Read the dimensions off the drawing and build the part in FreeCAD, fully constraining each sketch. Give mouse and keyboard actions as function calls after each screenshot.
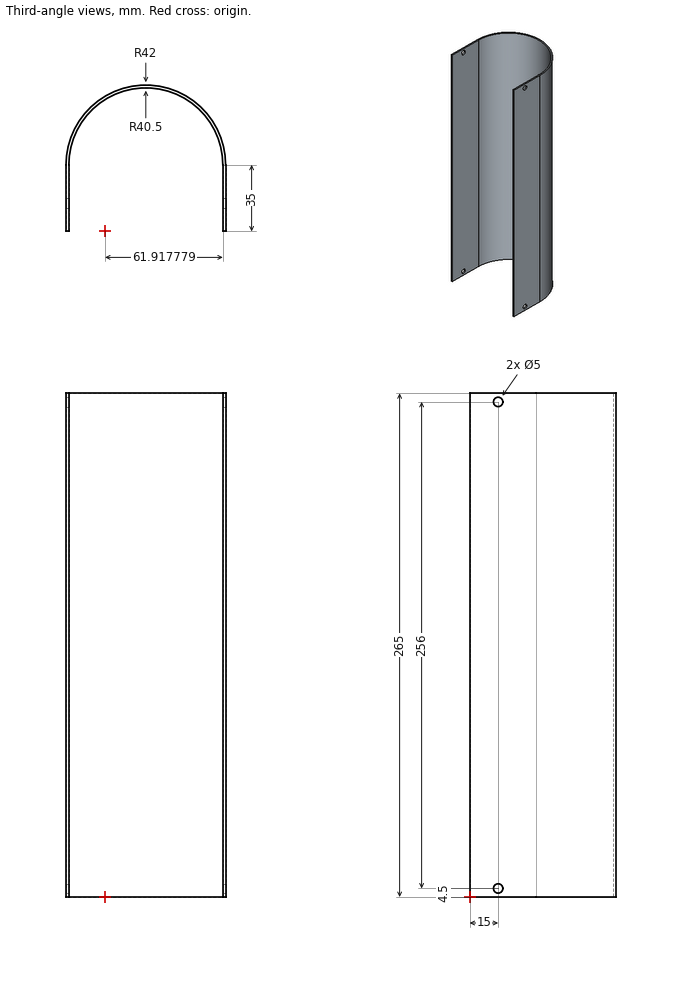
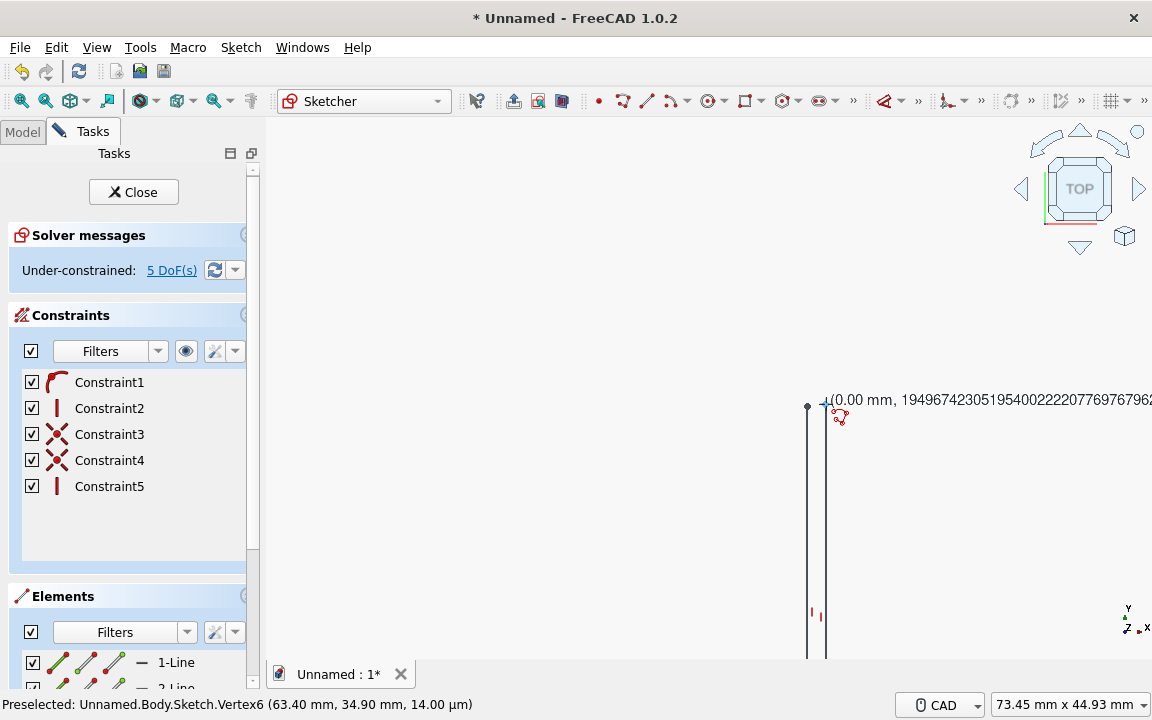
scroll(827, 403, down, 5)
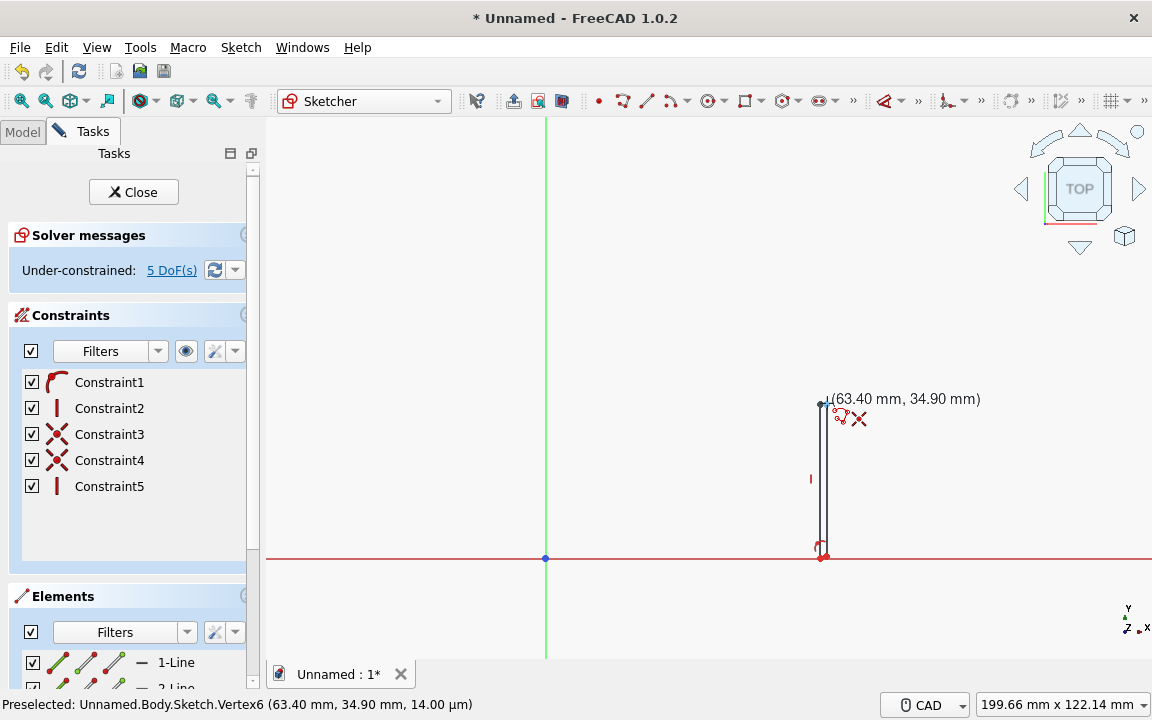
click(454, 404)
click(454, 559)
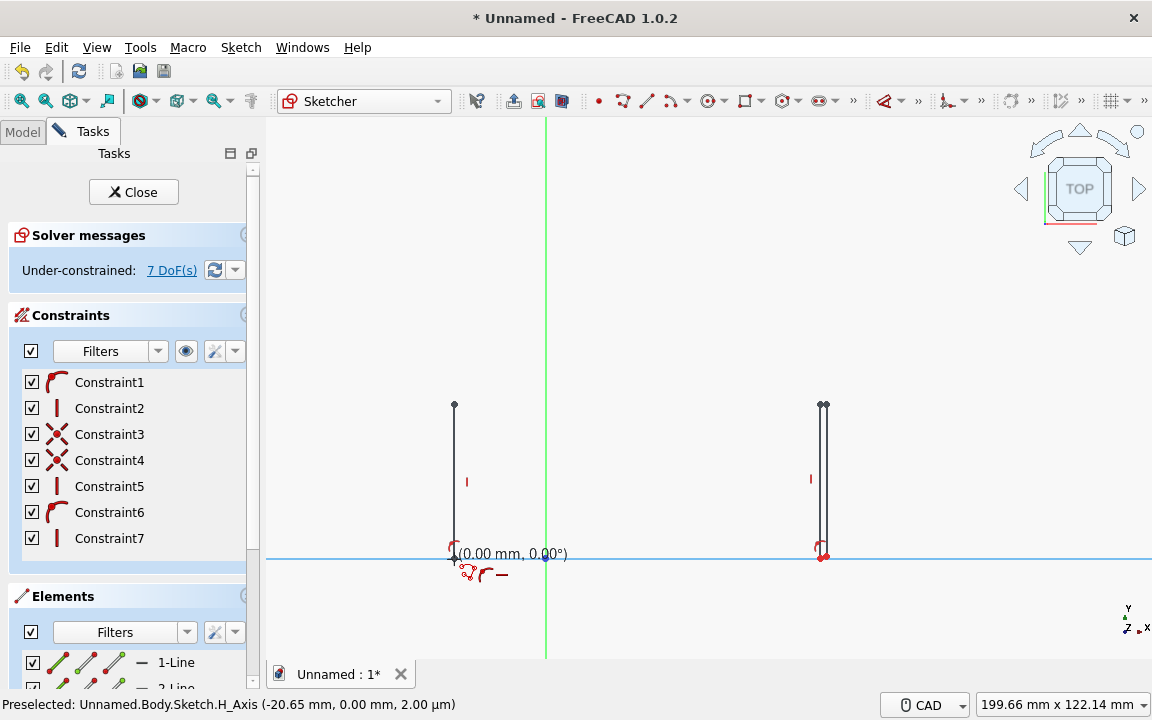
scroll(461, 559, up, 5)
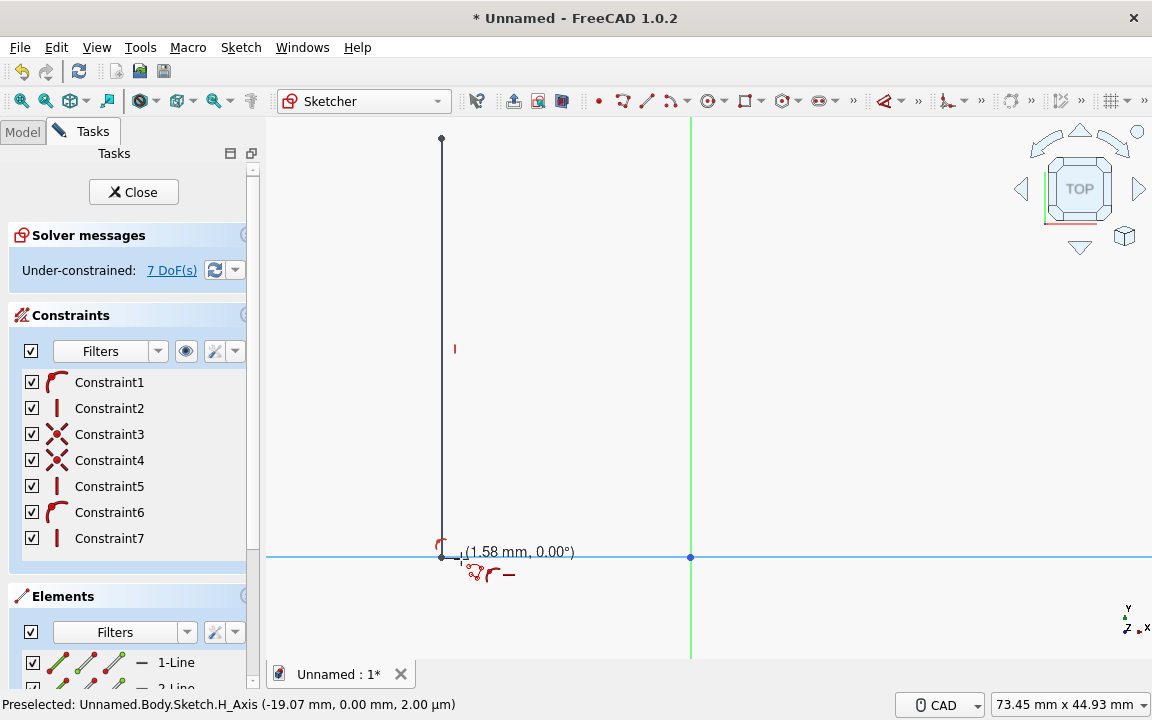
click(461, 548)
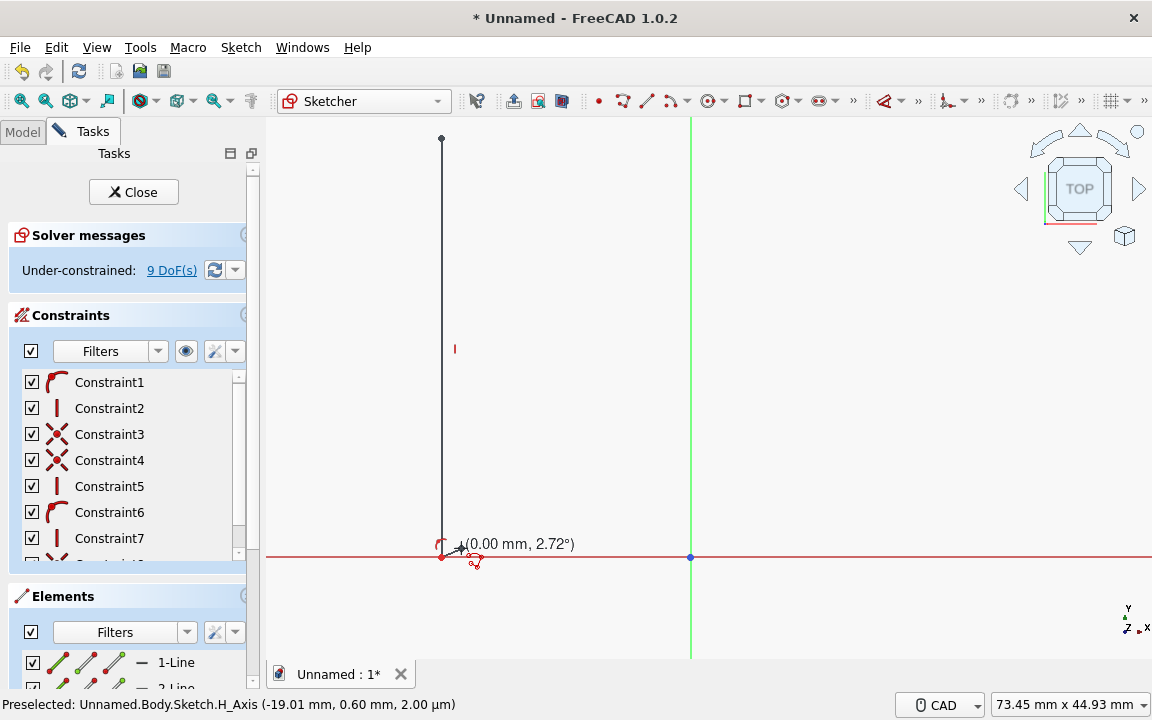
scroll(461, 560, down, 5)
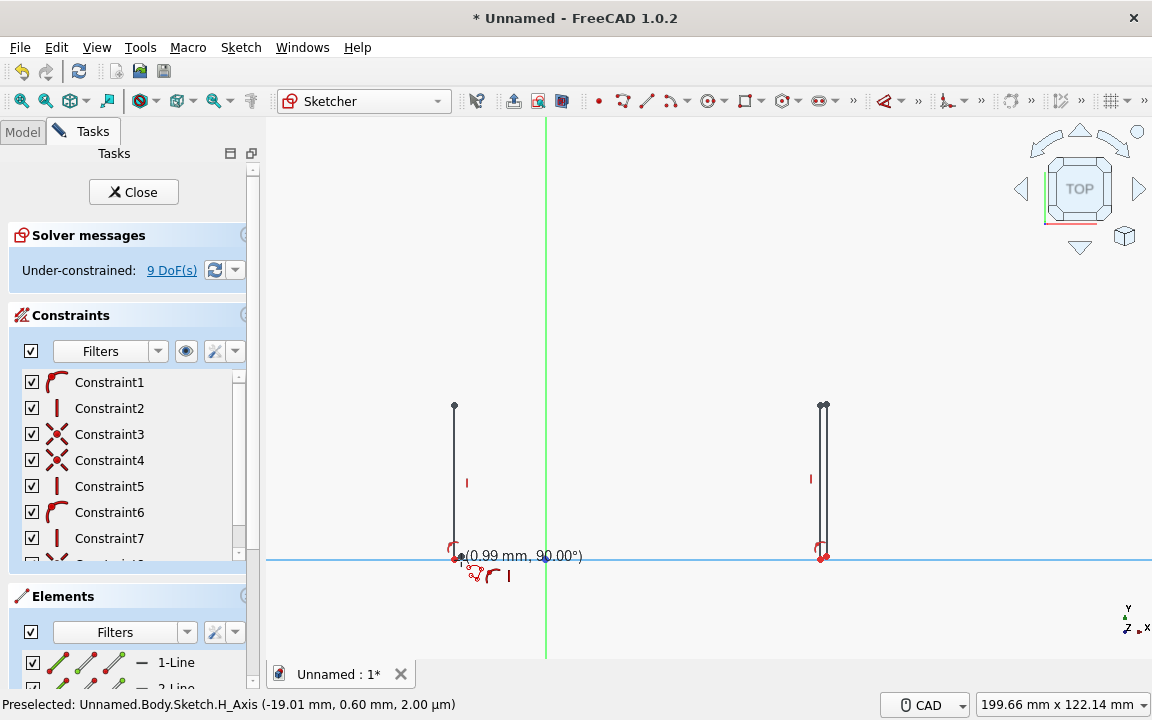
scroll(461, 404, up, 5)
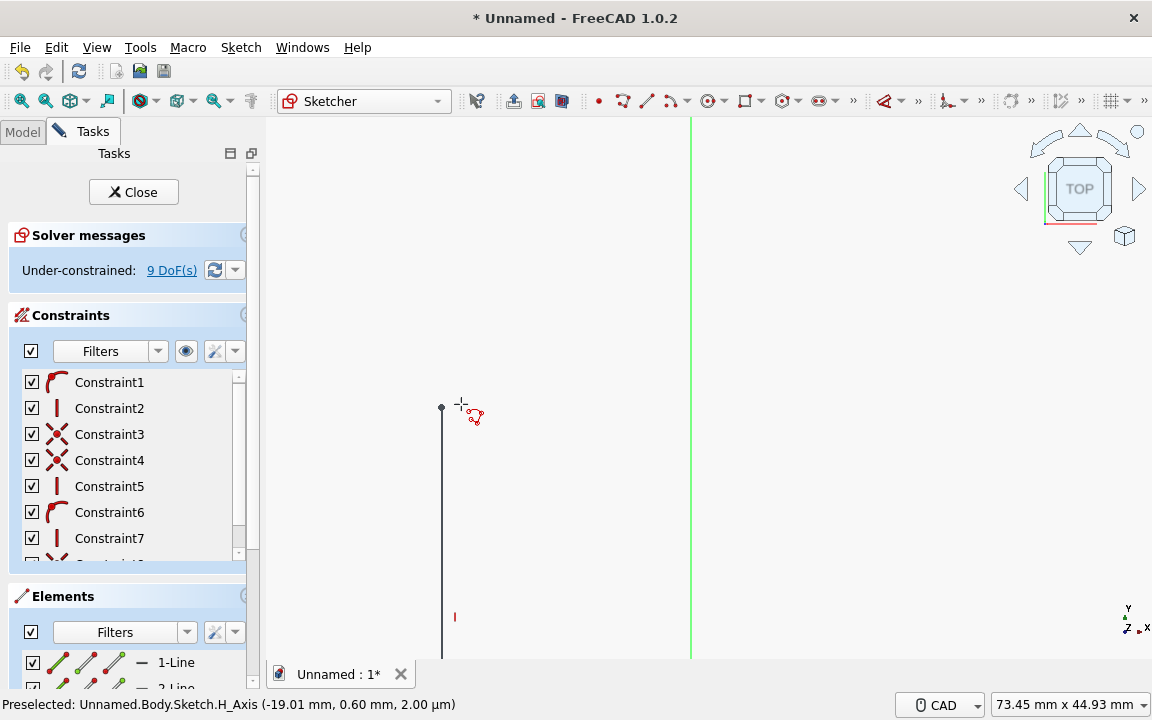
click(461, 404)
right_click(461, 404)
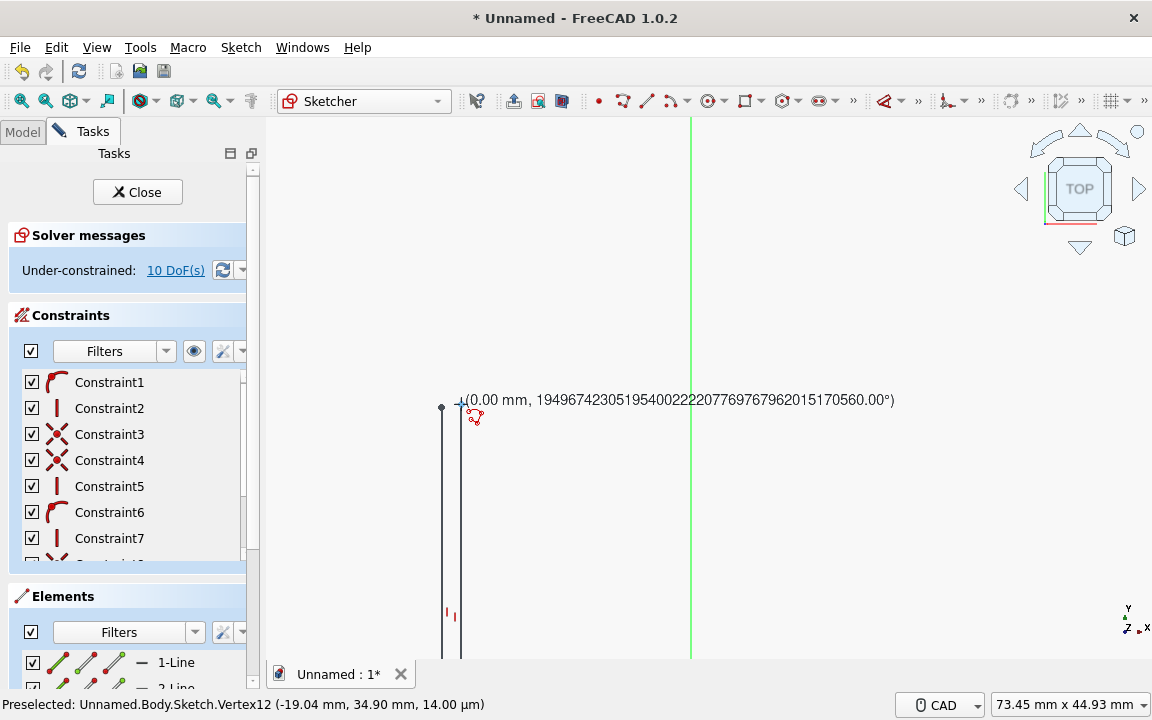
key(g)
key(3)
key(a)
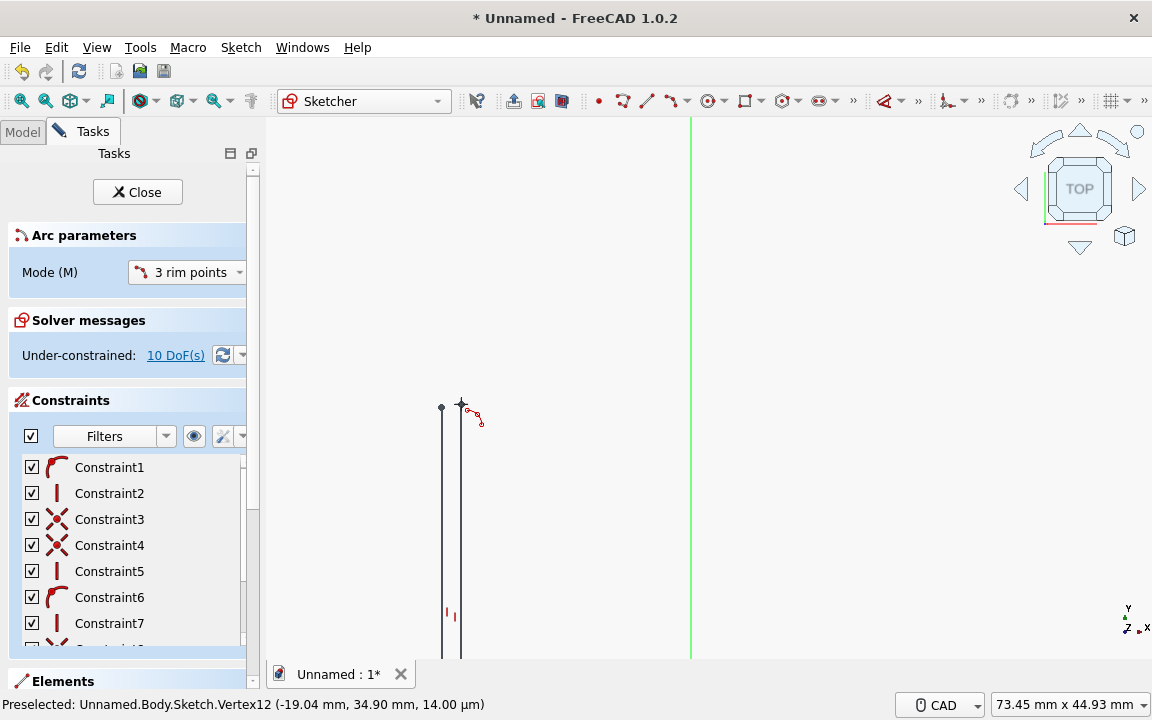
scroll(461, 403, down, 5)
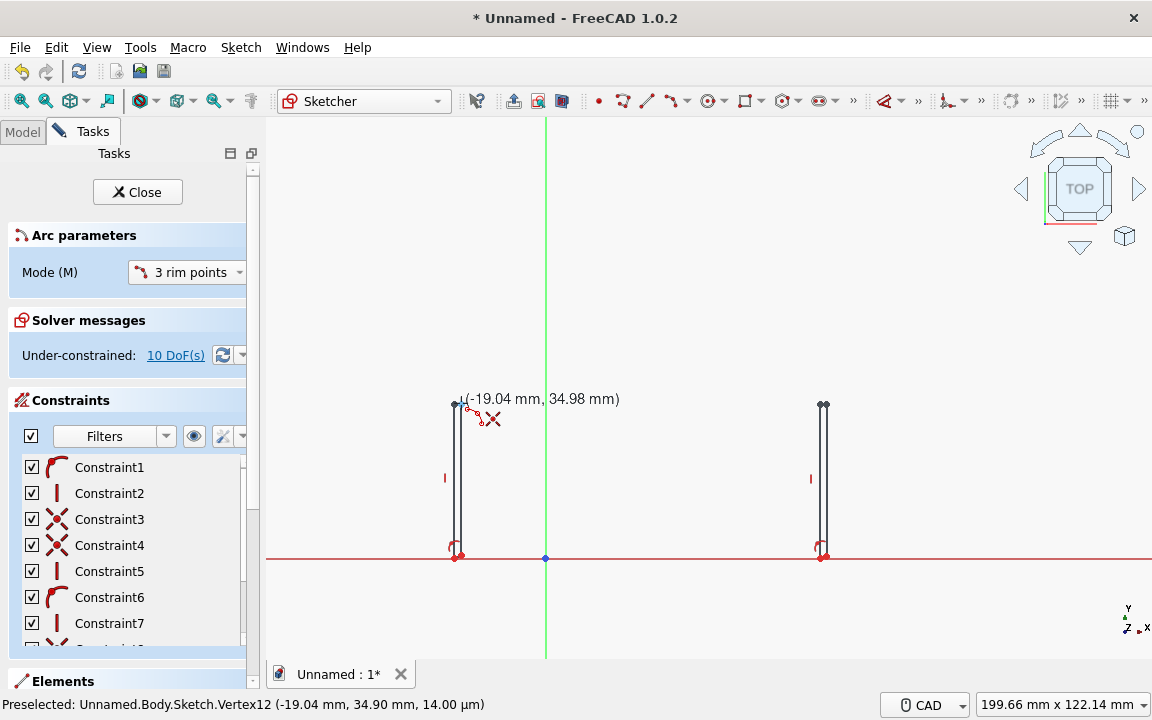
scroll(827, 404, up, 5)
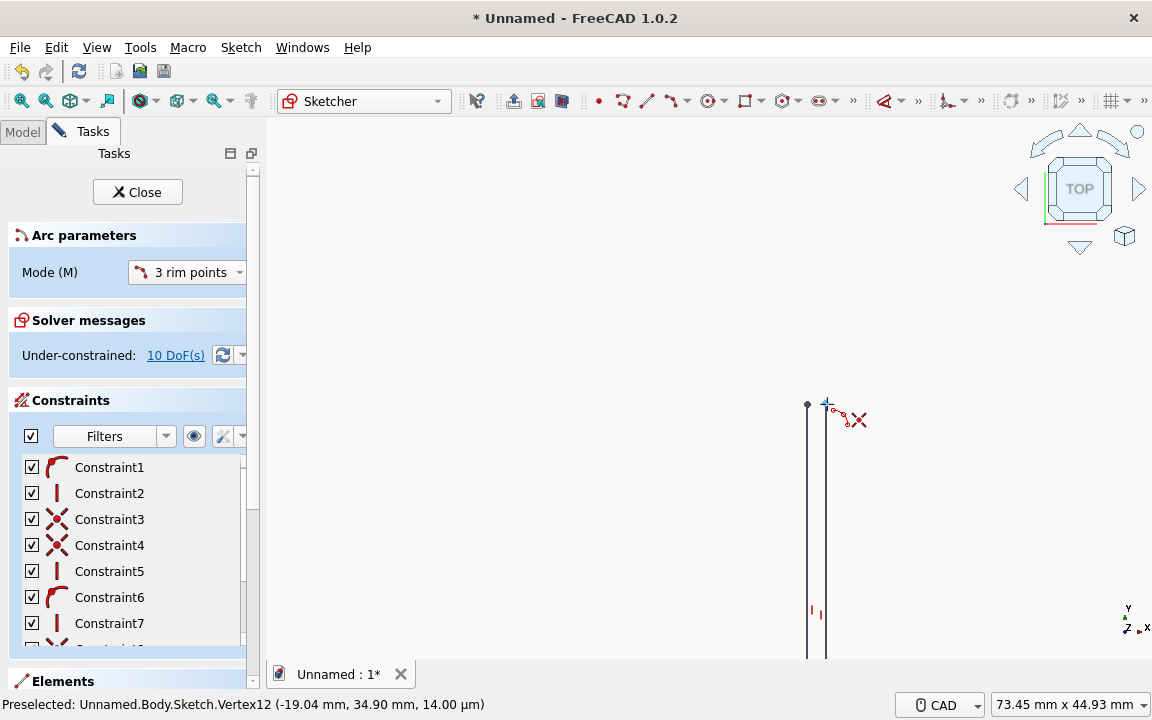
click(826, 403)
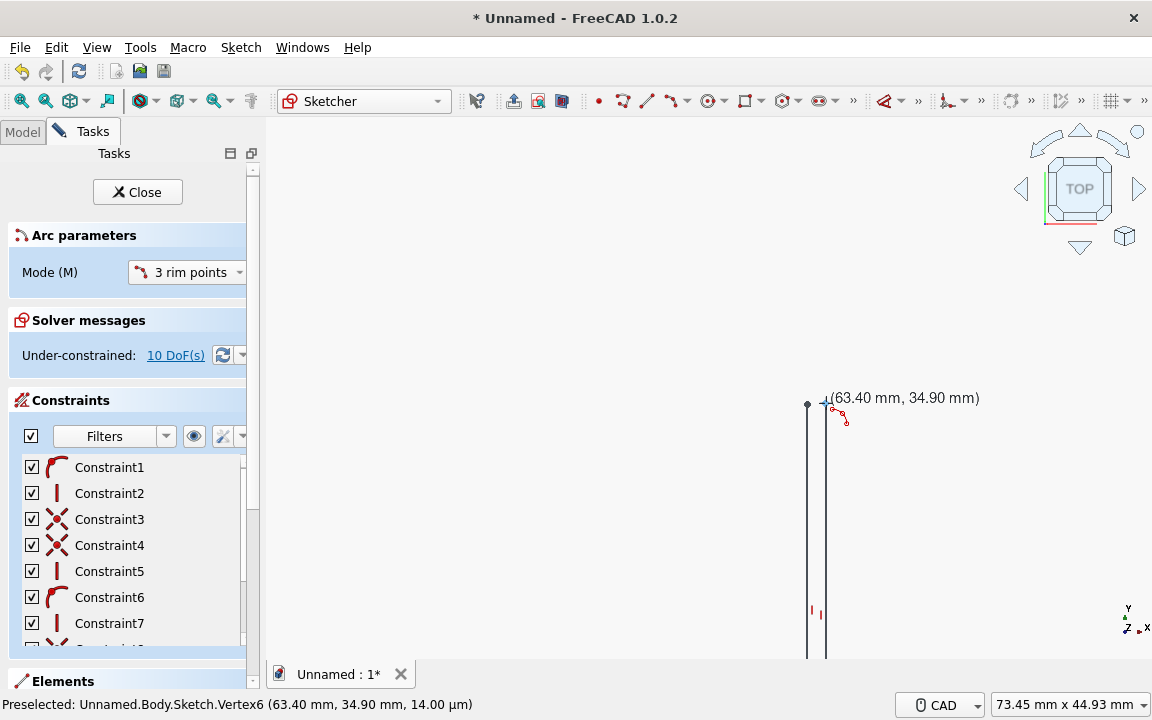
scroll(827, 404, down, 5)